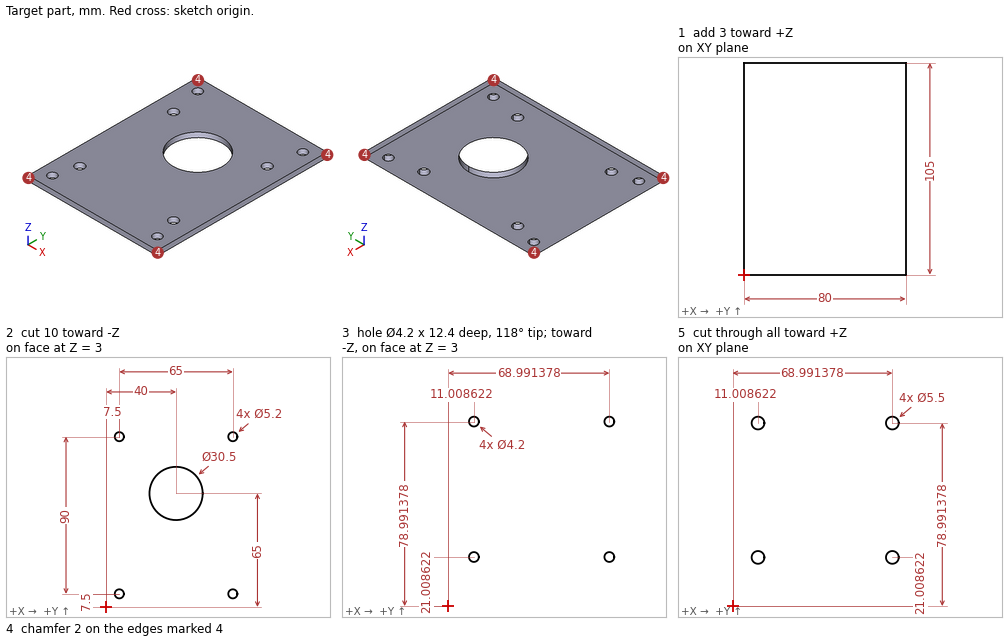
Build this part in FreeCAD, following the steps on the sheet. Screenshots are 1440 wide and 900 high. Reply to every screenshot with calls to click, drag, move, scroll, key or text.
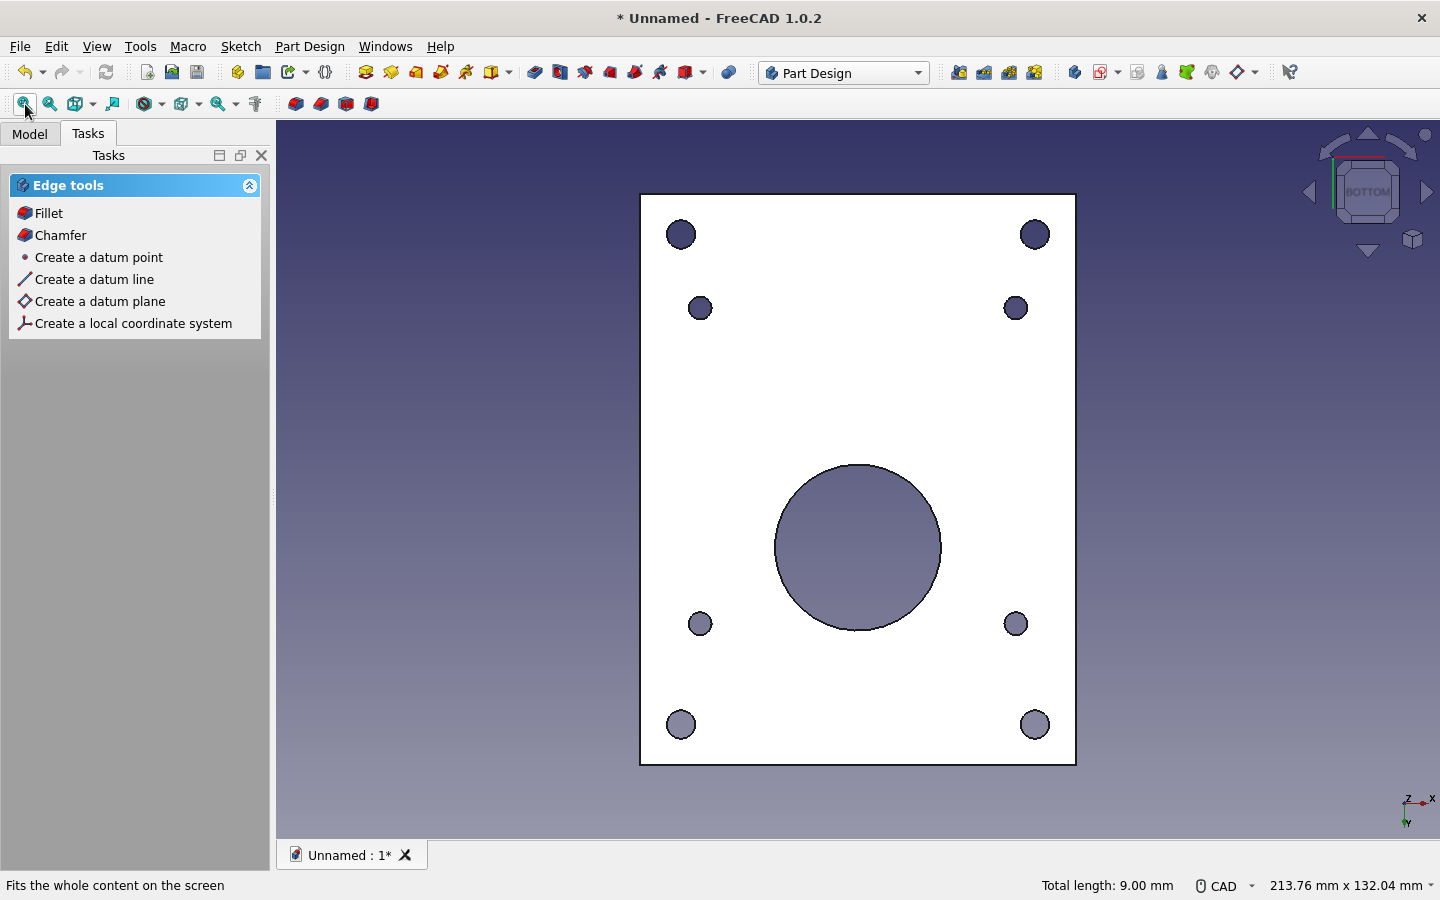
scroll(640, 764, up, 5)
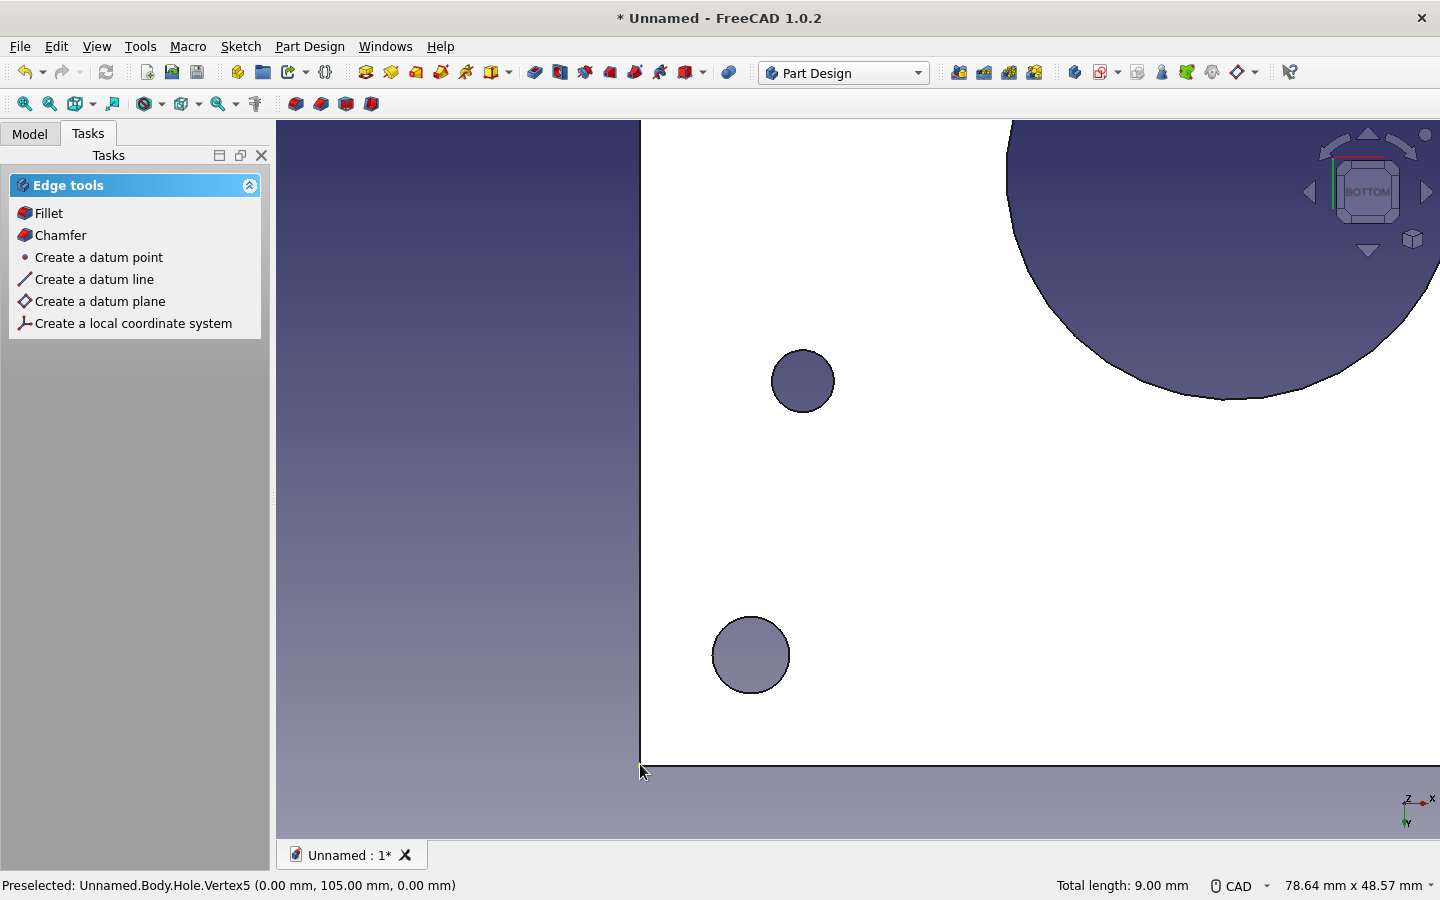
click(25, 104)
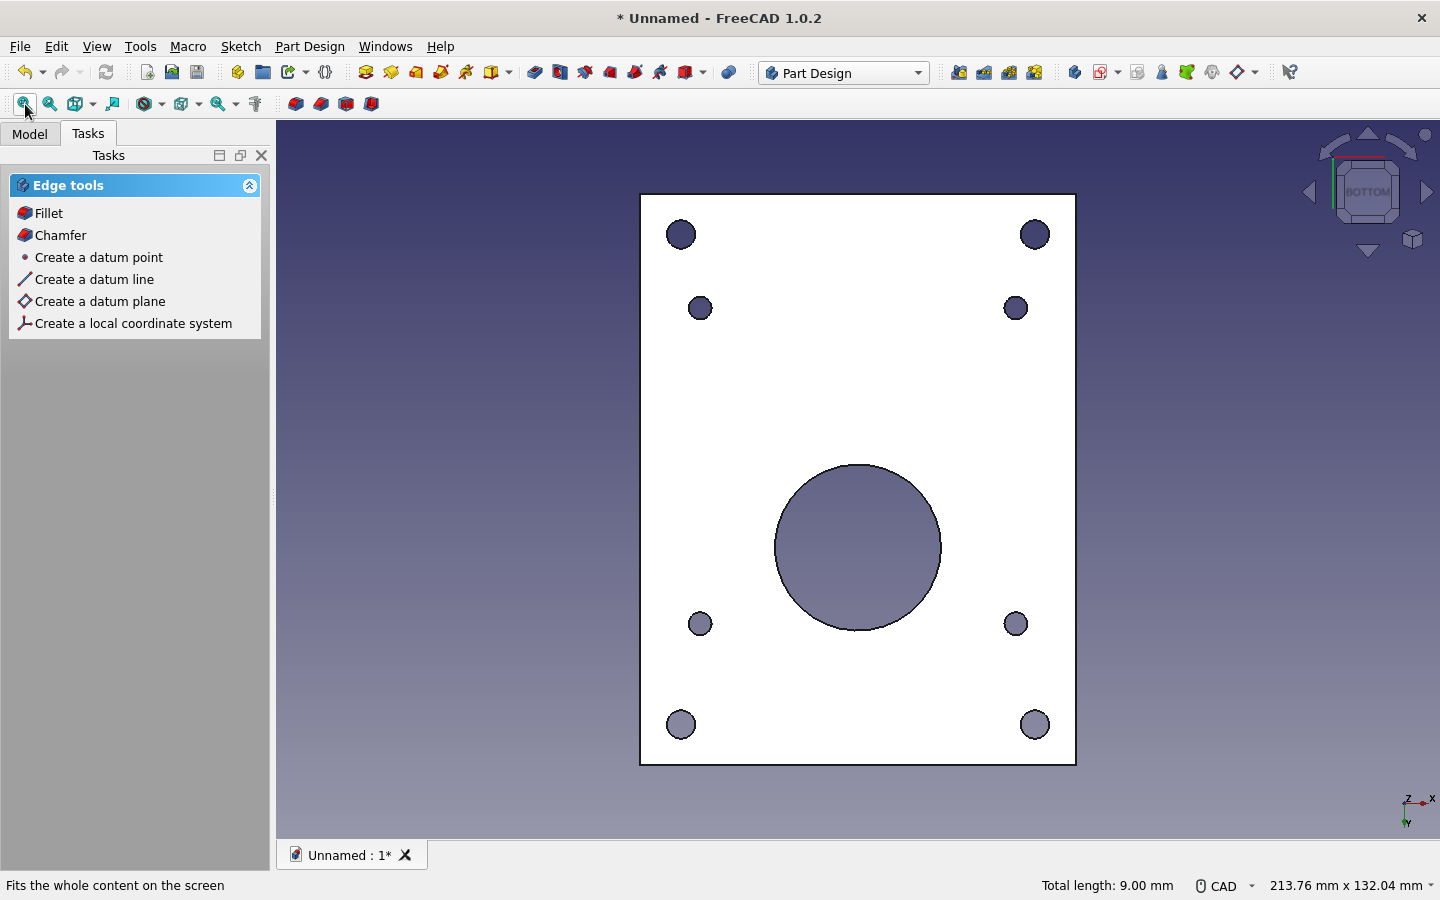
key(4)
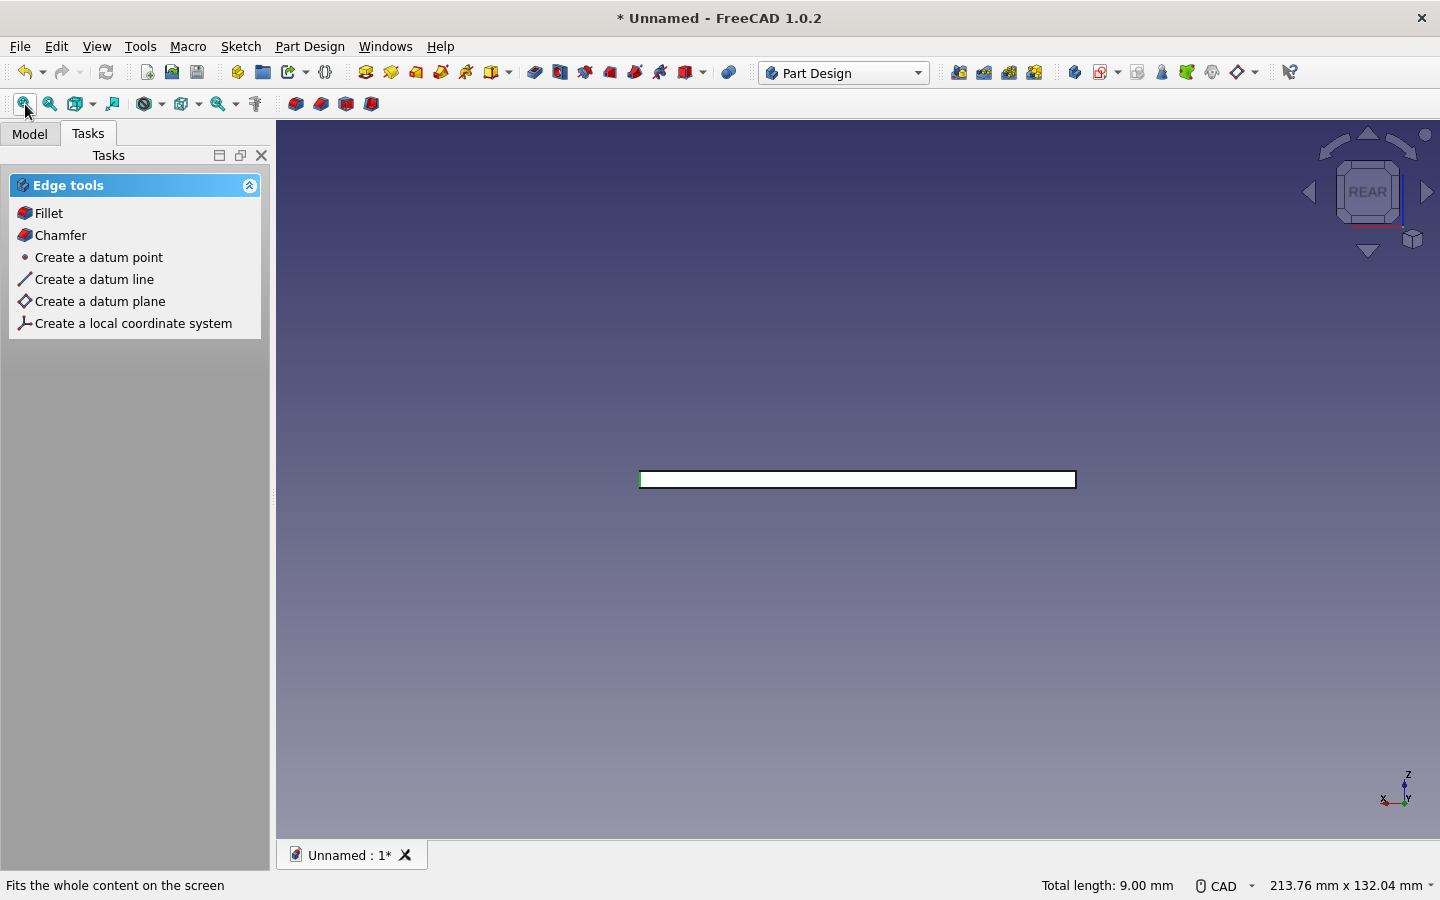
click(25, 104)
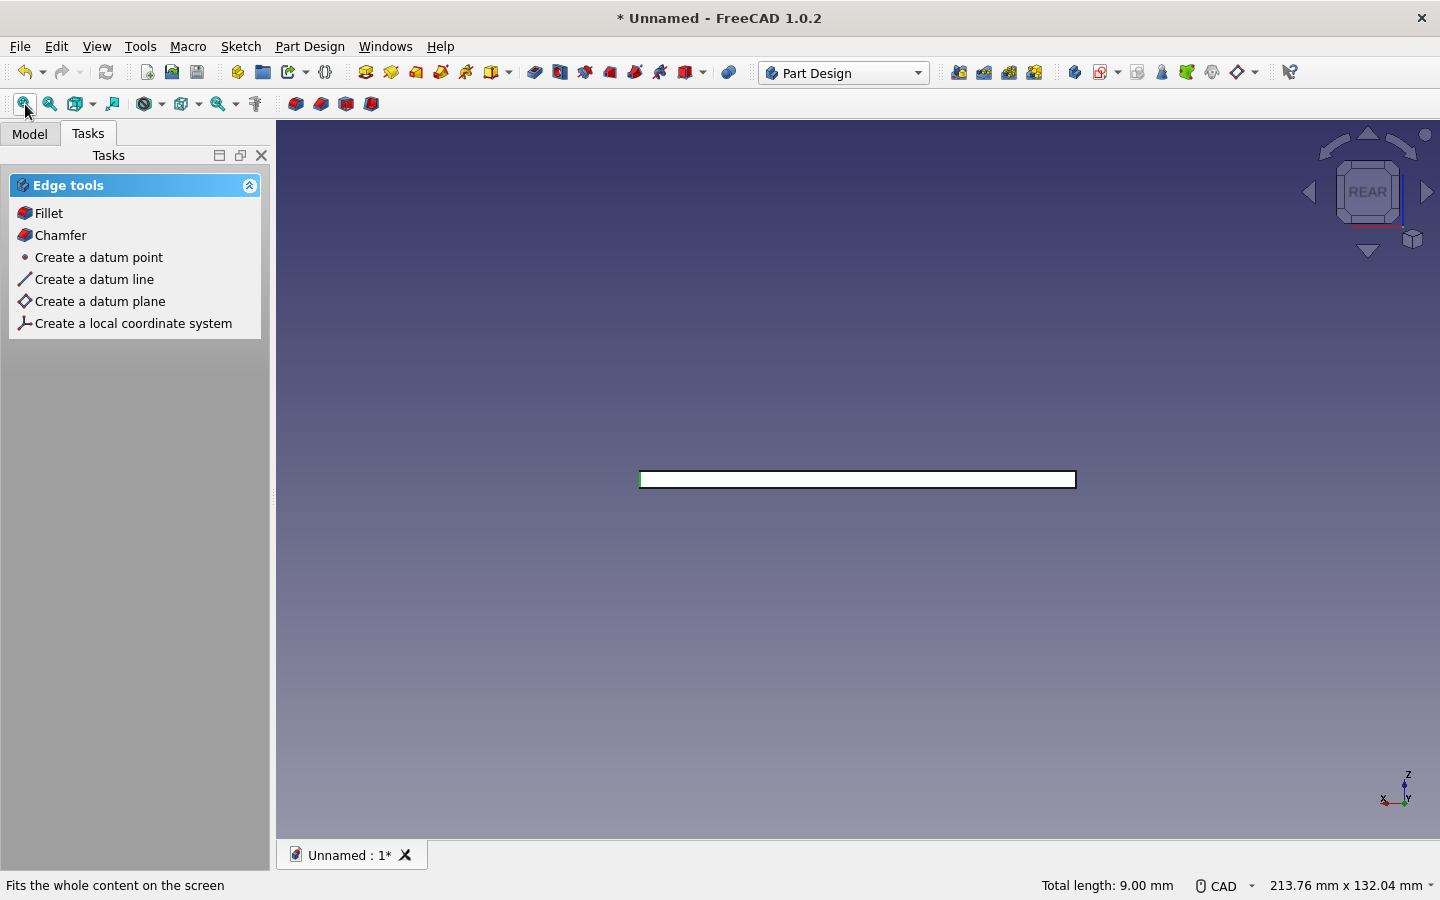
click(1076, 479, ctrl)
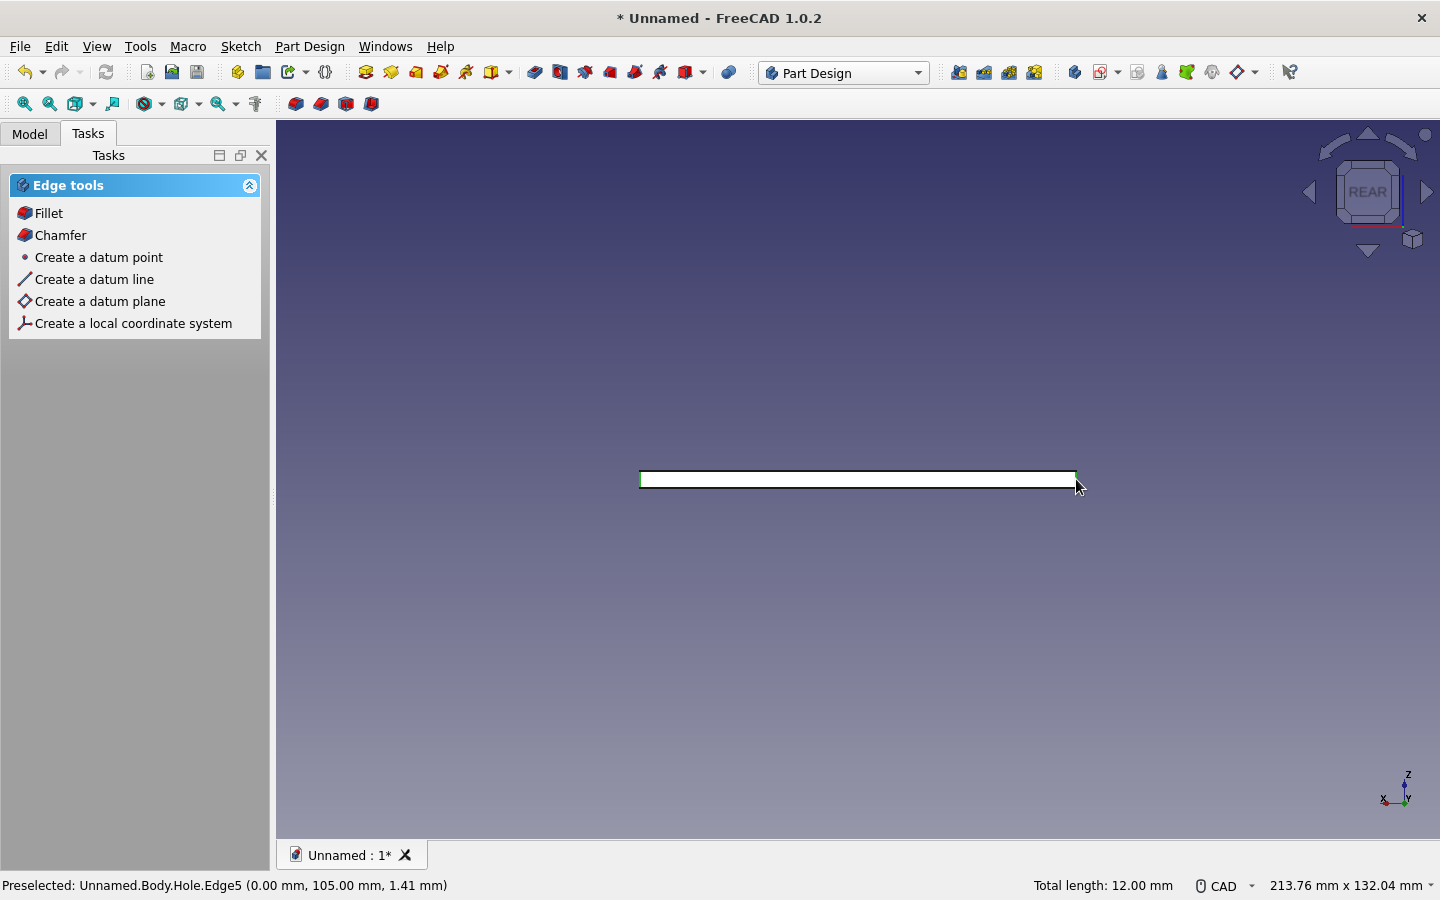
click(321, 104)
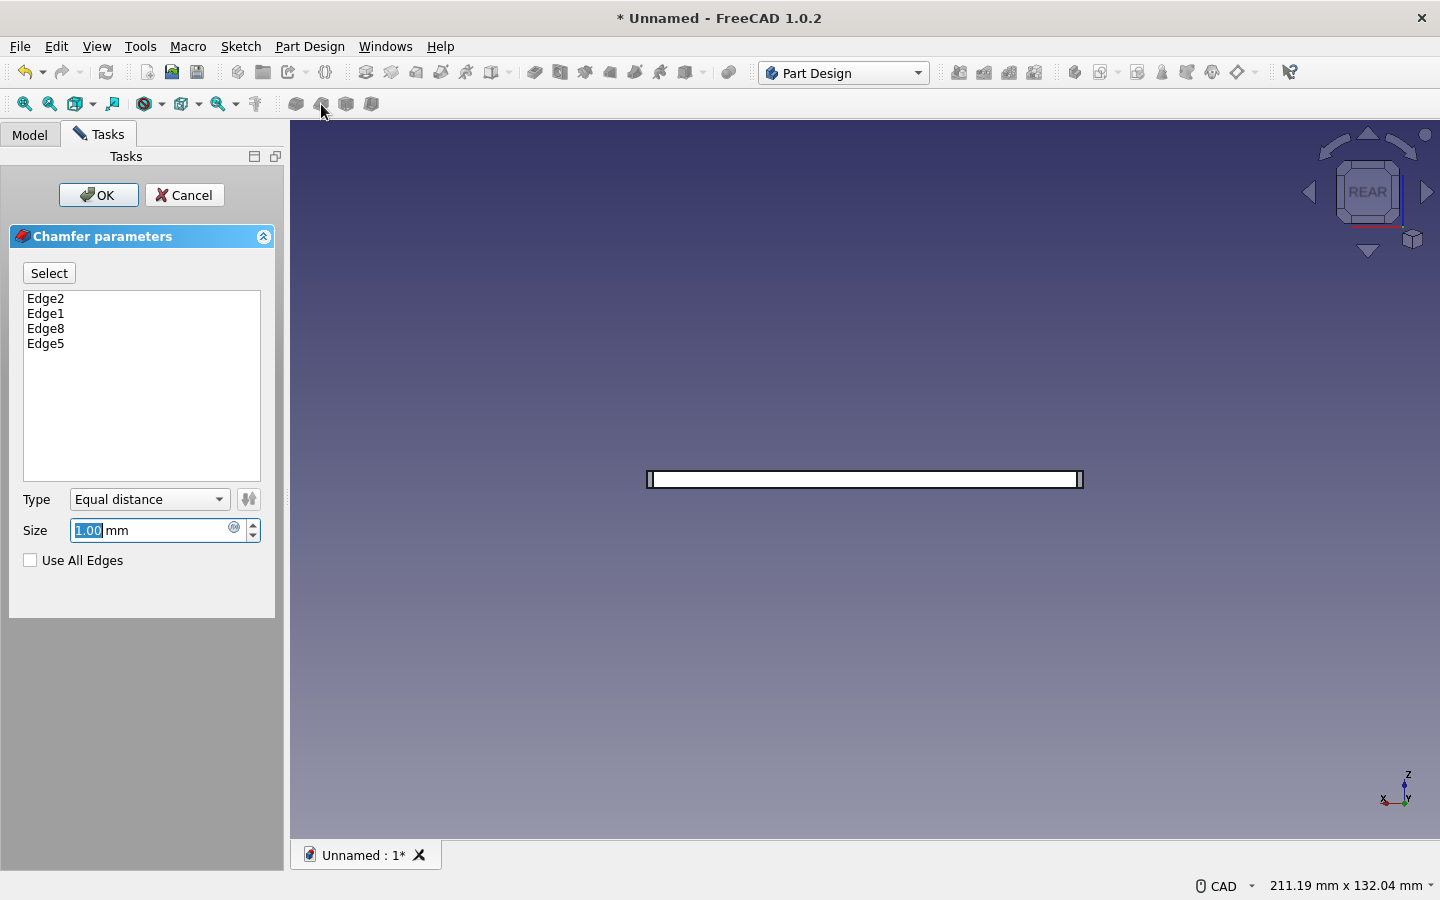
text(2)
key(Tab)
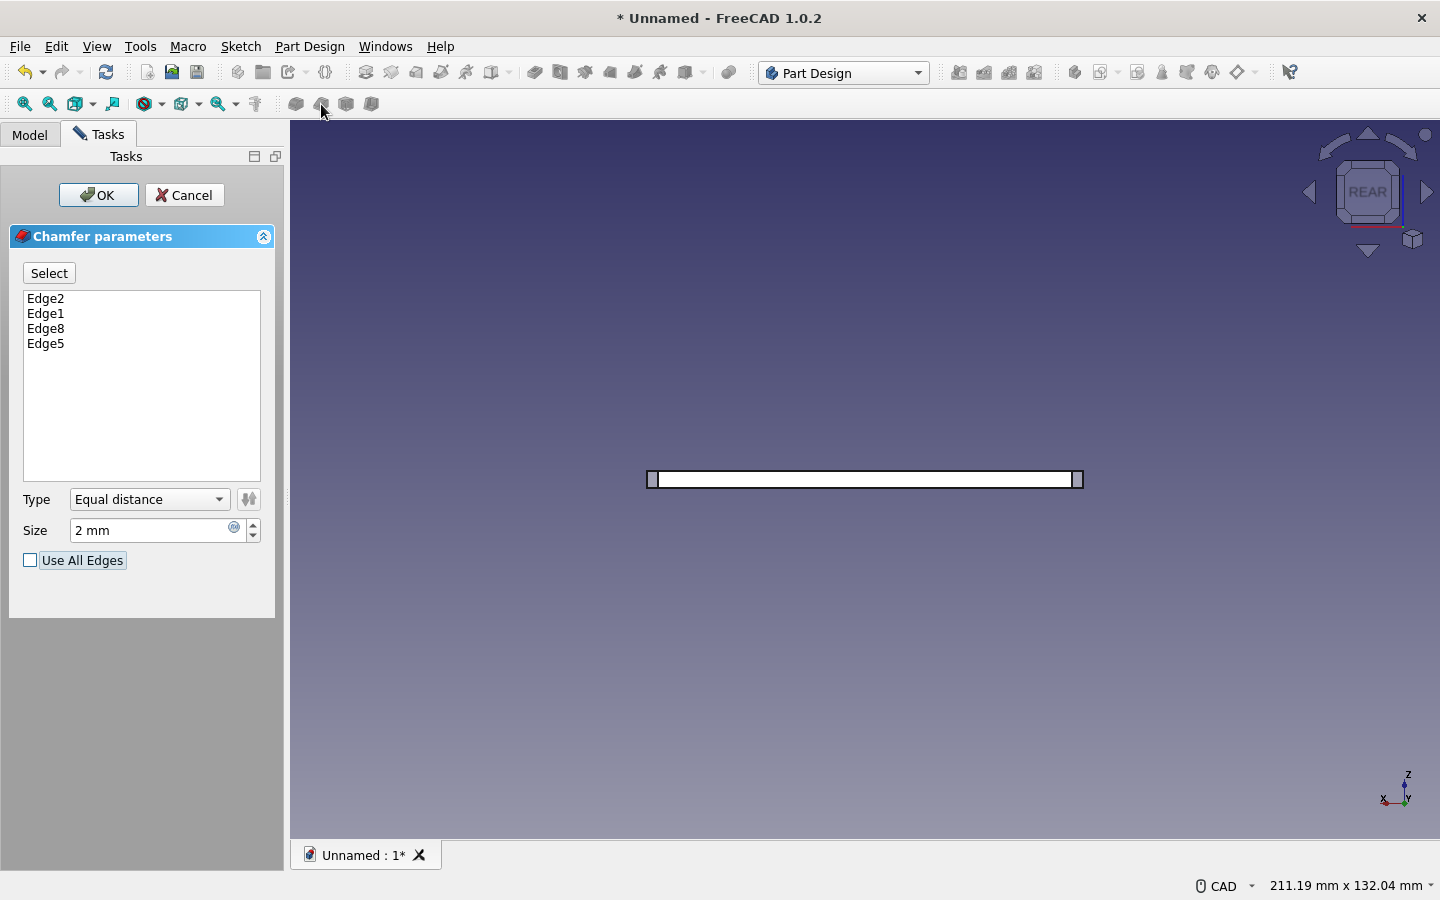
click(99, 195)